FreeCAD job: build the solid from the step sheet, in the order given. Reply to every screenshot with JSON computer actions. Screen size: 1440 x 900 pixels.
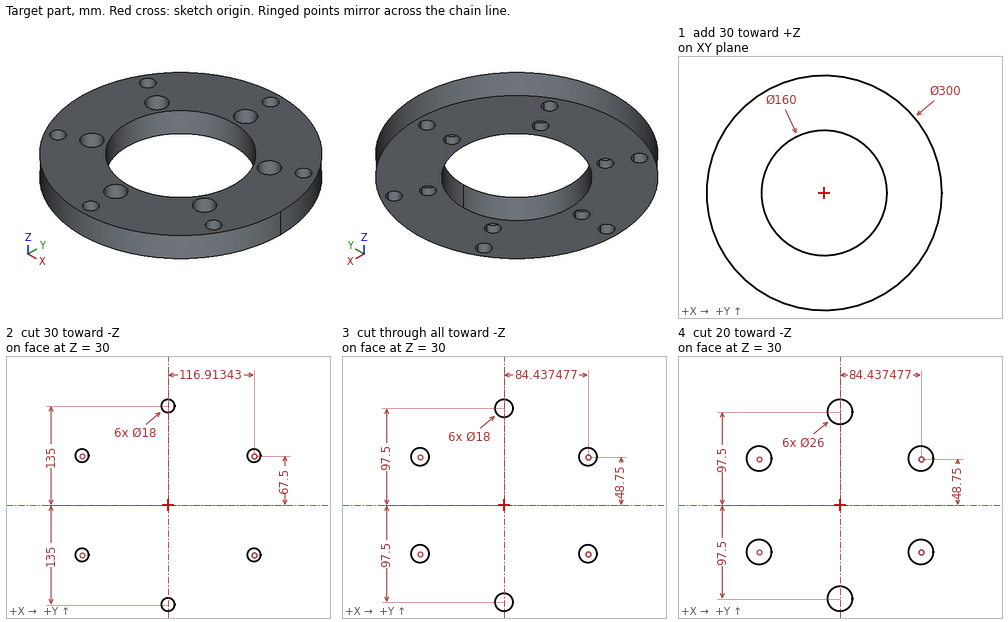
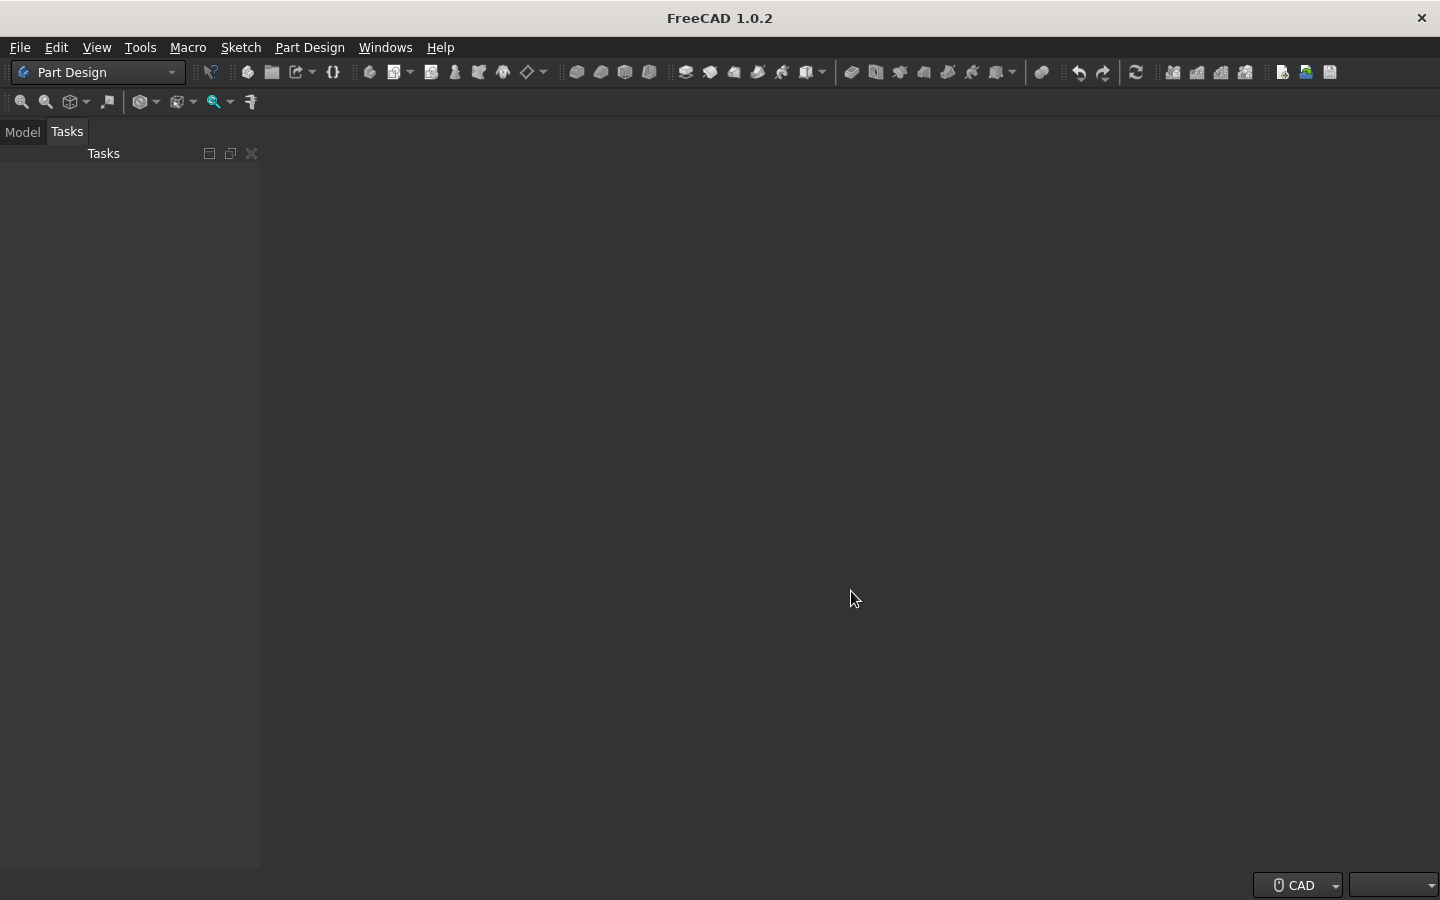
{"action": "key", "text": "ctrl+n"}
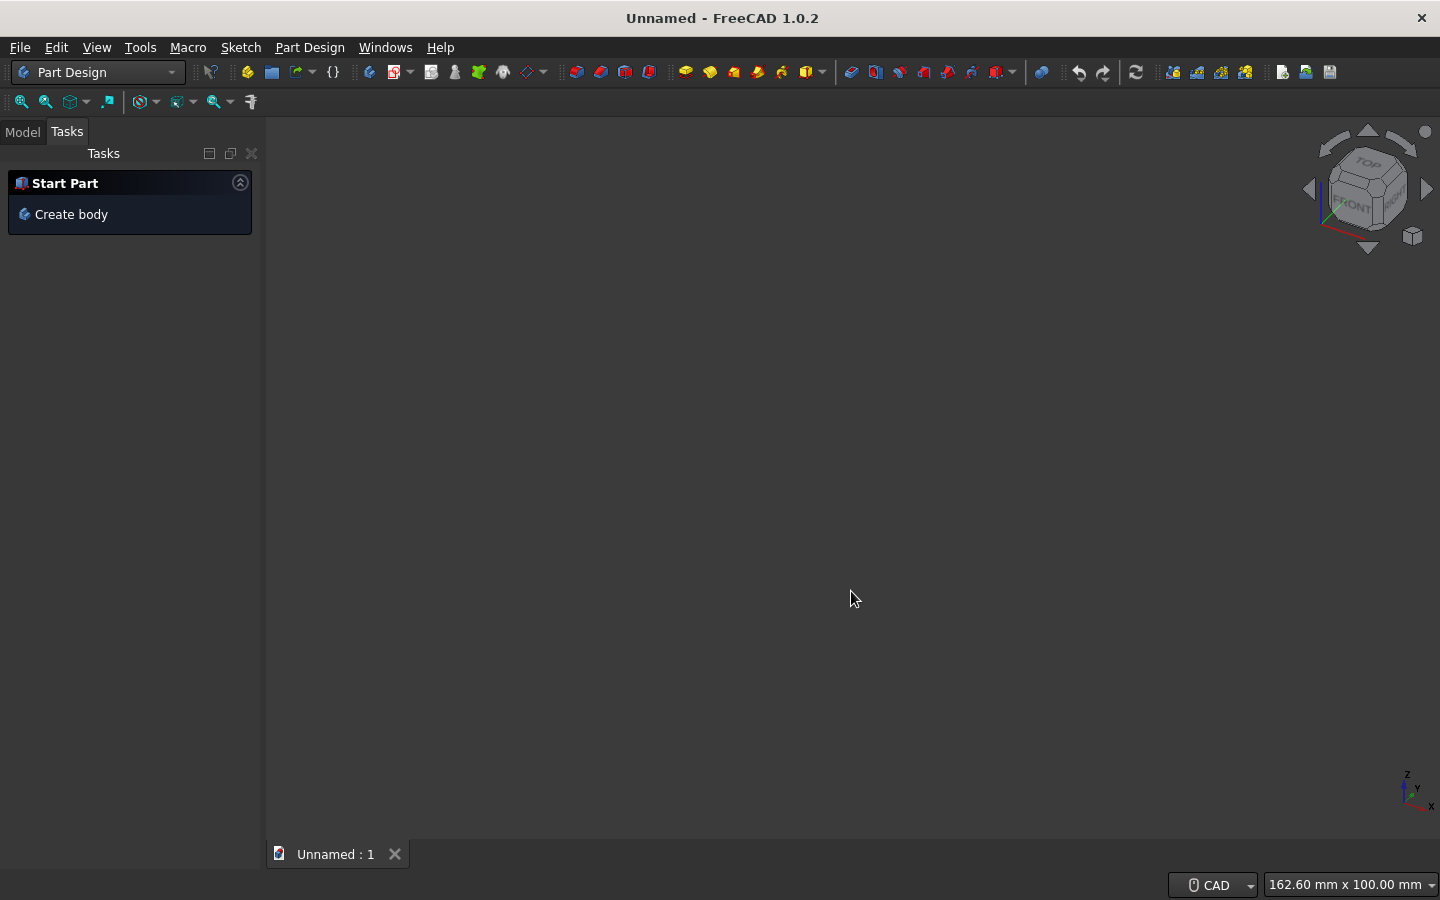
{"action": "left_click", "coordinate": [394, 72]}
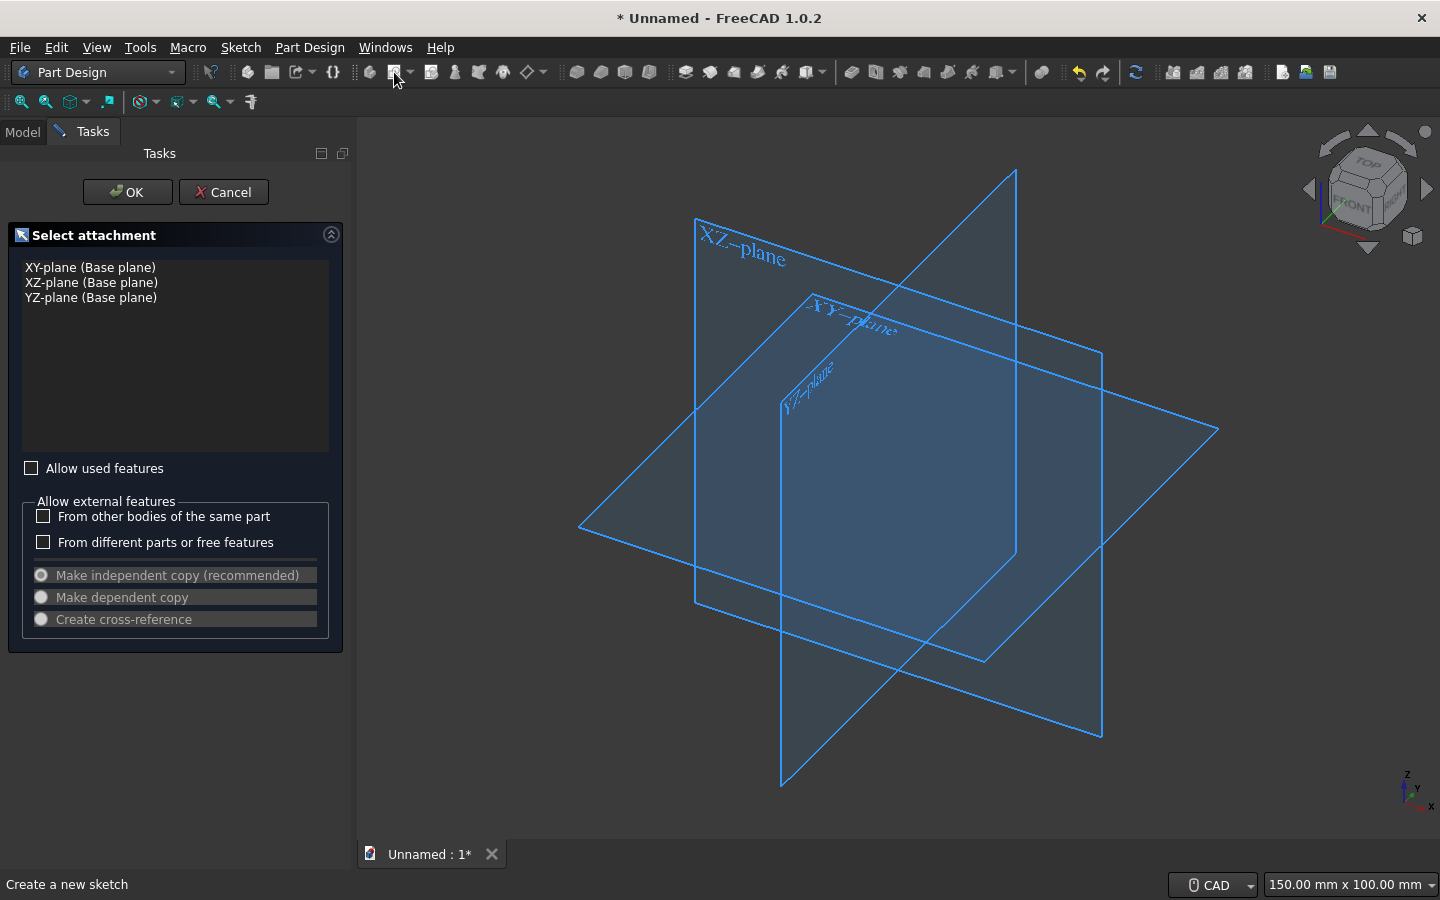
{"action": "left_click", "coordinate": [82, 268]}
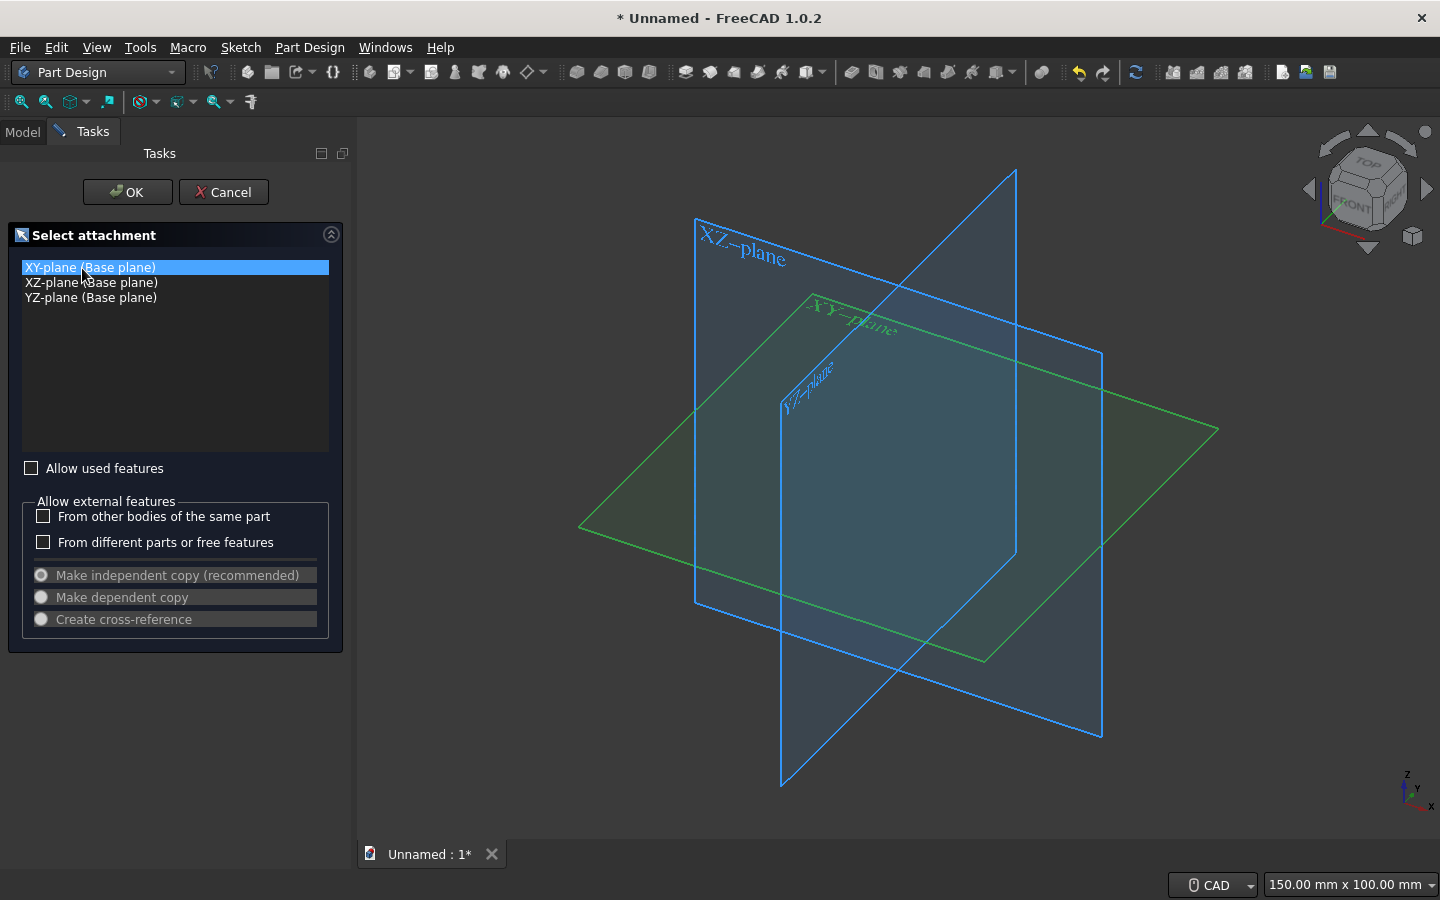
{"action": "left_click", "coordinate": [128, 192]}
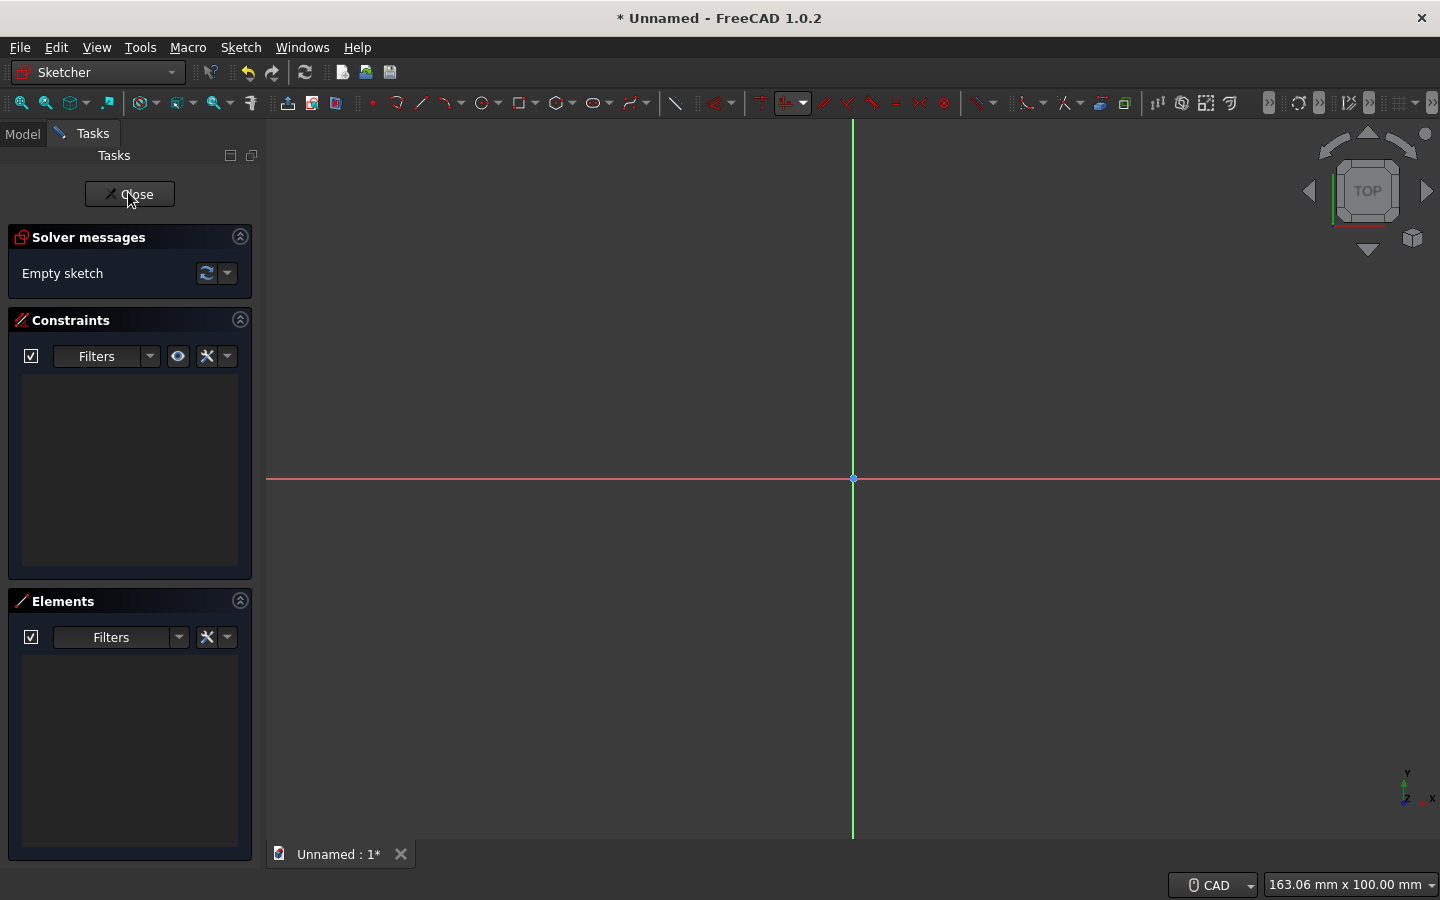
{"action": "scroll", "coordinate": [767, 479], "scroll_direction": "down", "scroll_amount": 8}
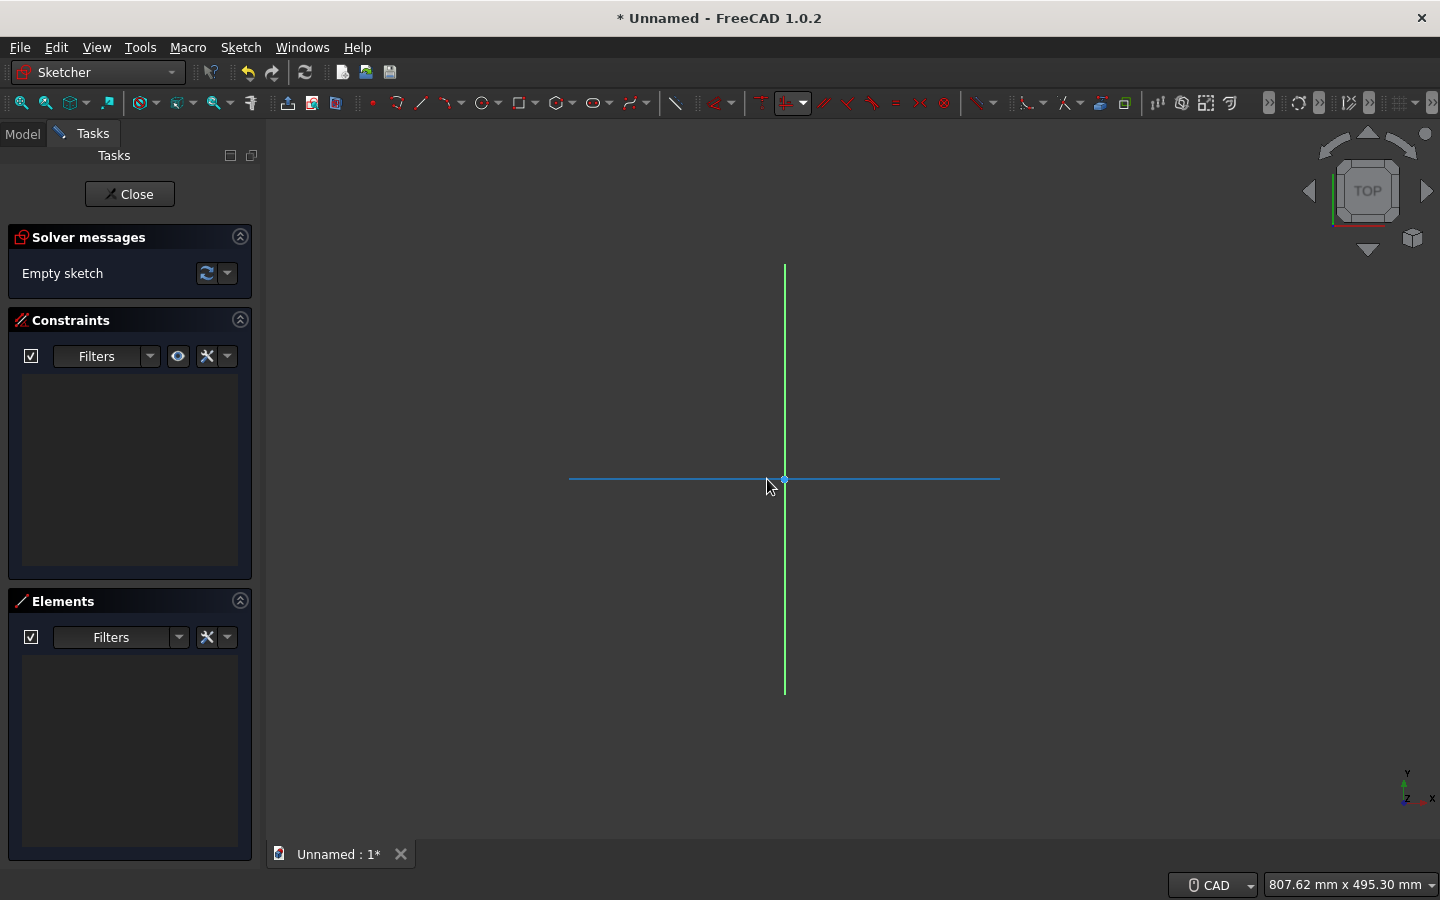
{"action": "left_click", "coordinate": [482, 104]}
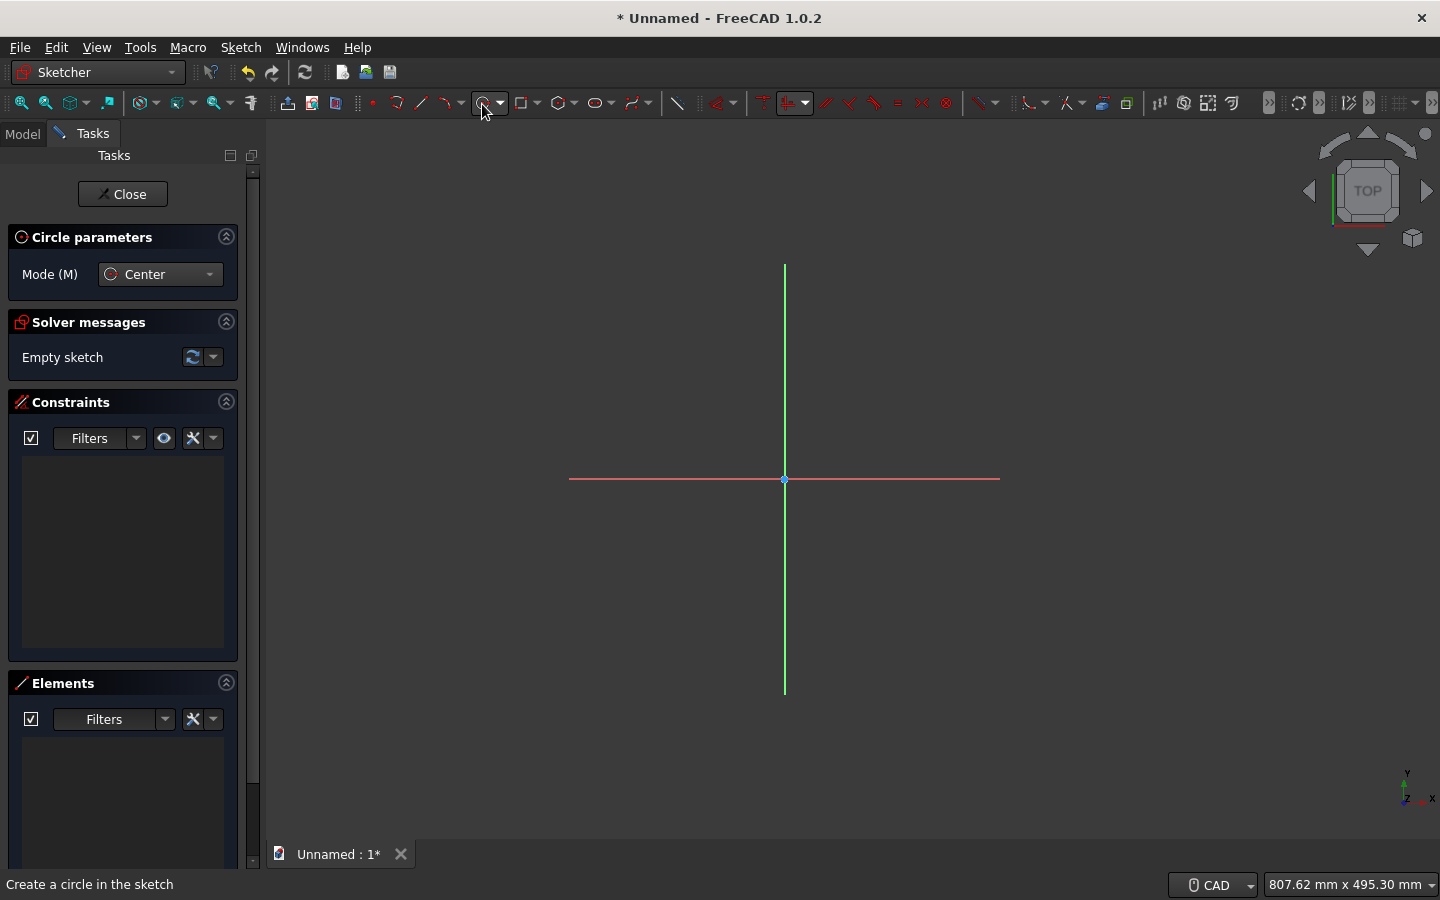
{"action": "left_click", "coordinate": [785, 479]}
{"action": "left_click", "coordinate": [939, 325]}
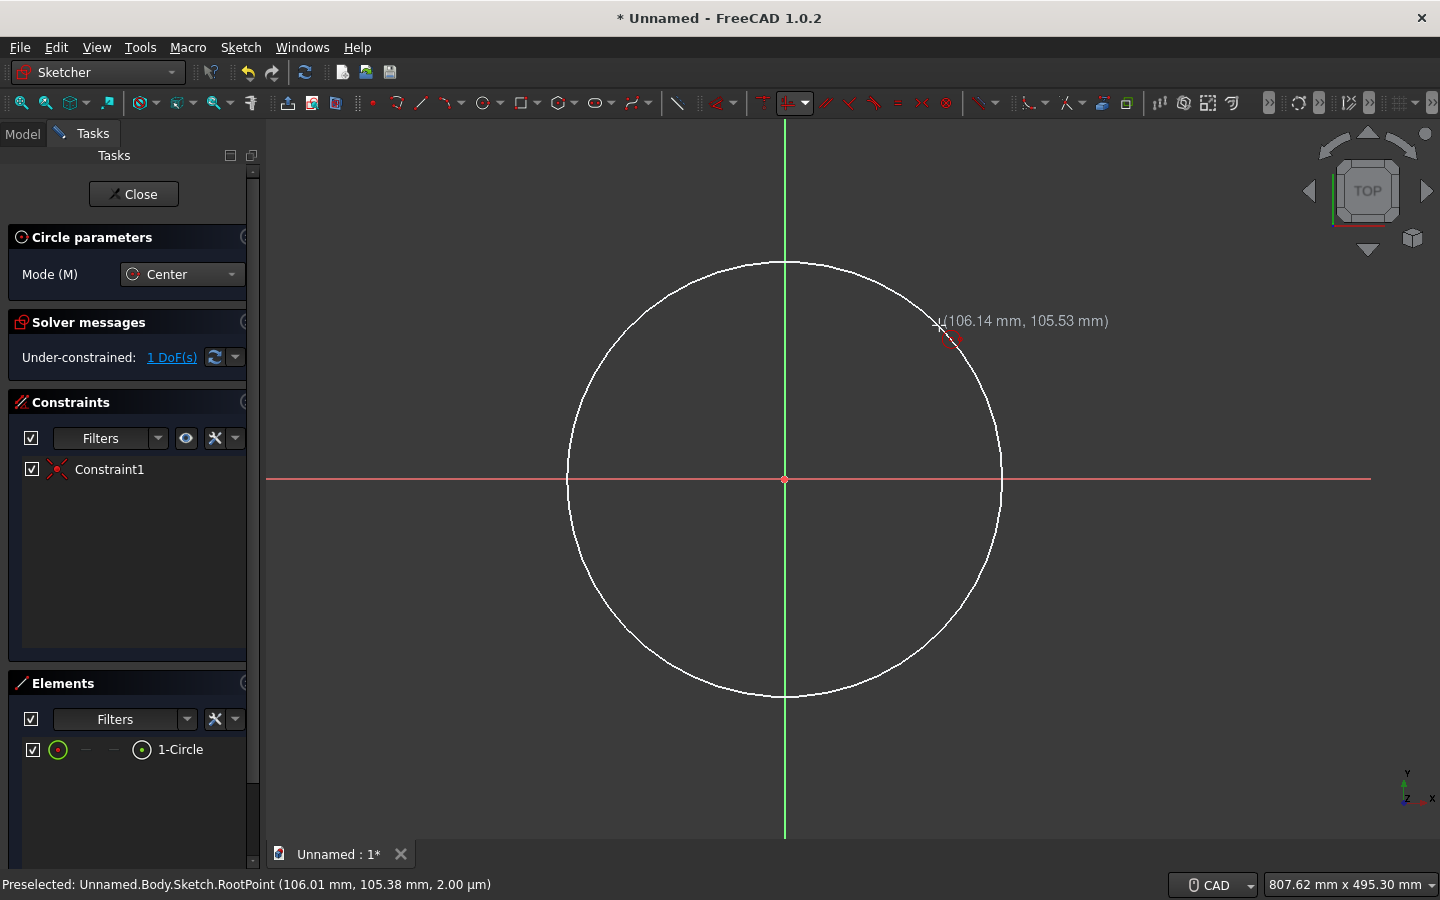
{"action": "left_click", "coordinate": [785, 479]}
{"action": "left_click", "coordinate": [867, 397]}
{"action": "key", "text": "Escape"}